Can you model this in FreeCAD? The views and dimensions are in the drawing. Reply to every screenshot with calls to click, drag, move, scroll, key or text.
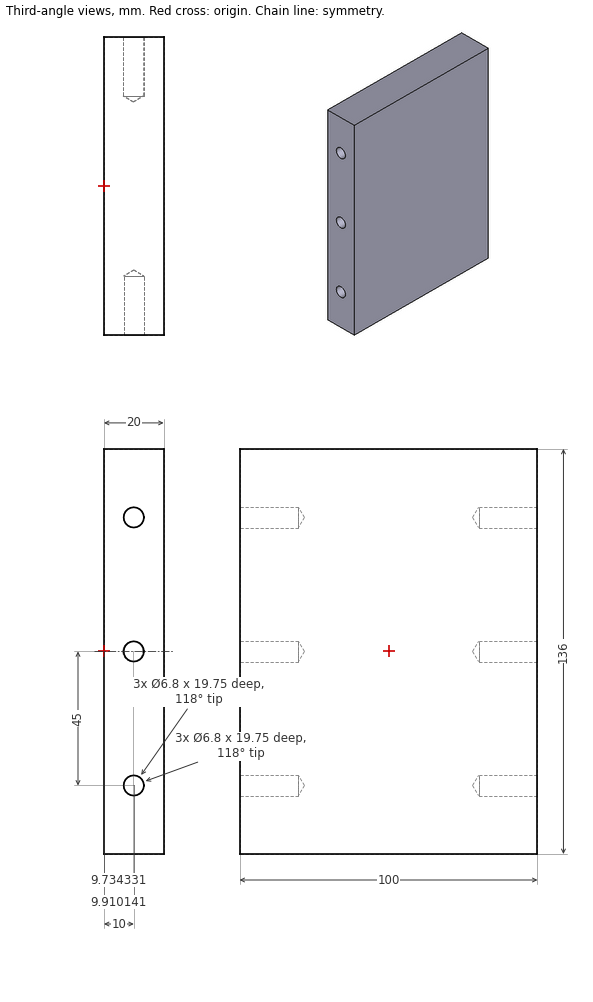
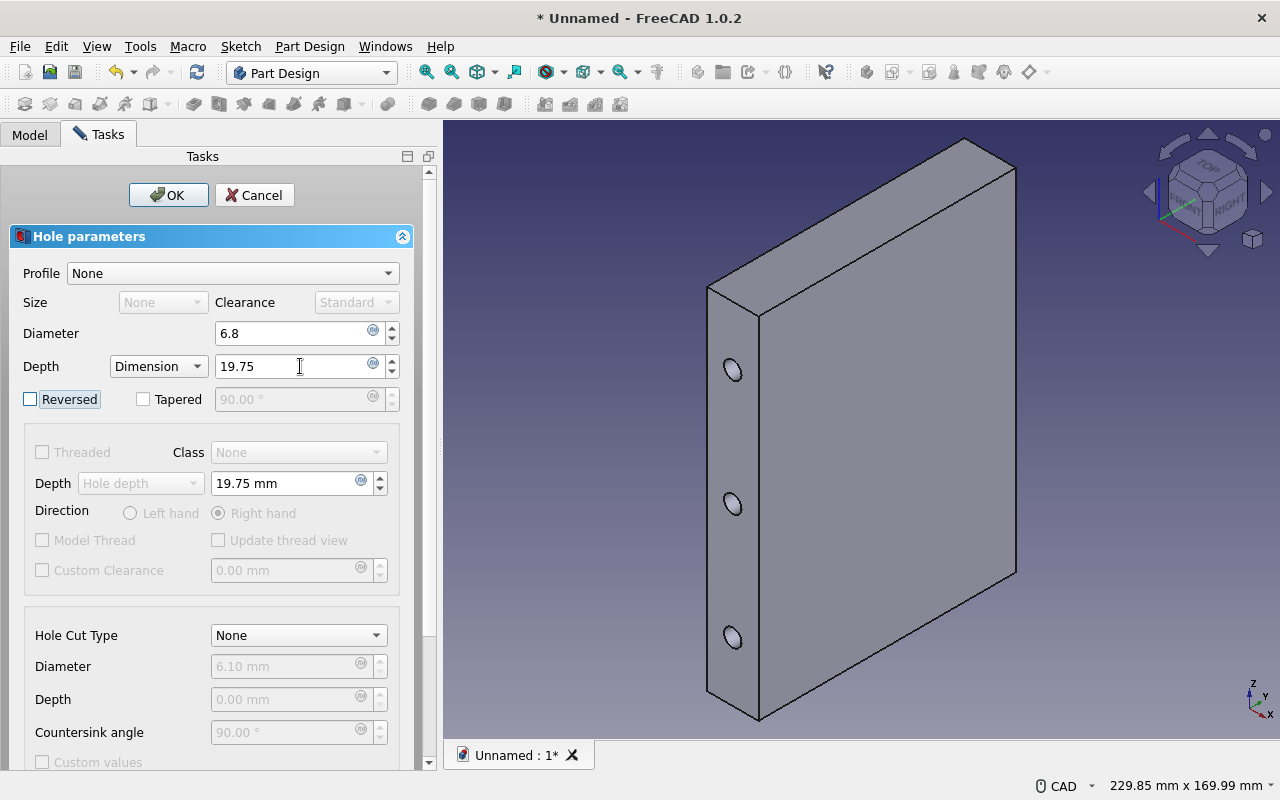
click(169, 195)